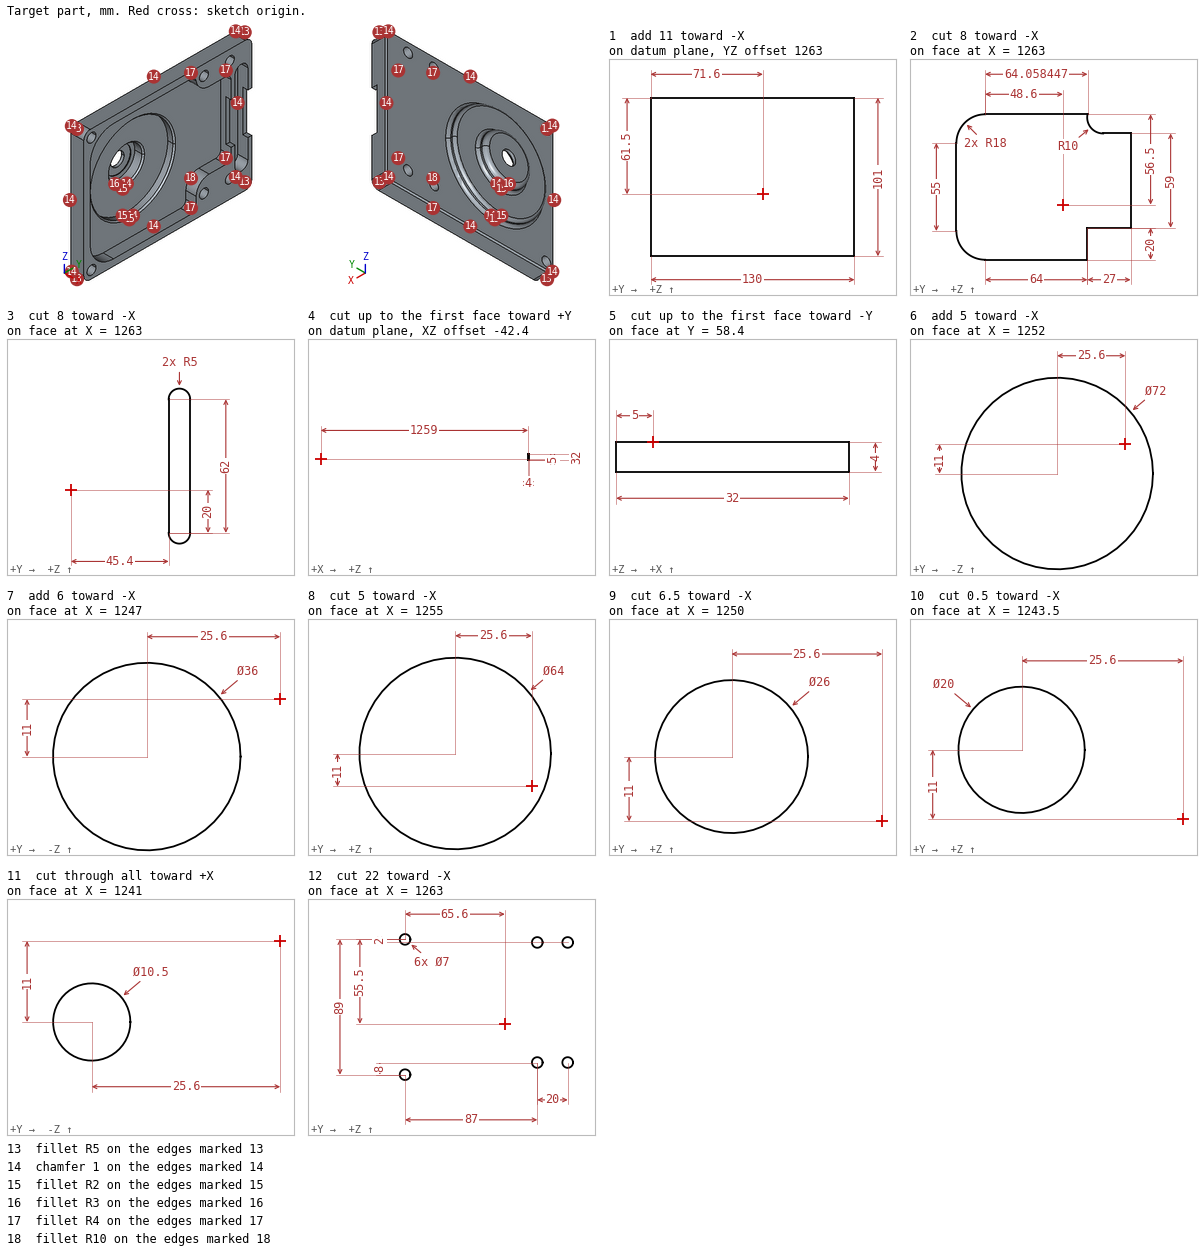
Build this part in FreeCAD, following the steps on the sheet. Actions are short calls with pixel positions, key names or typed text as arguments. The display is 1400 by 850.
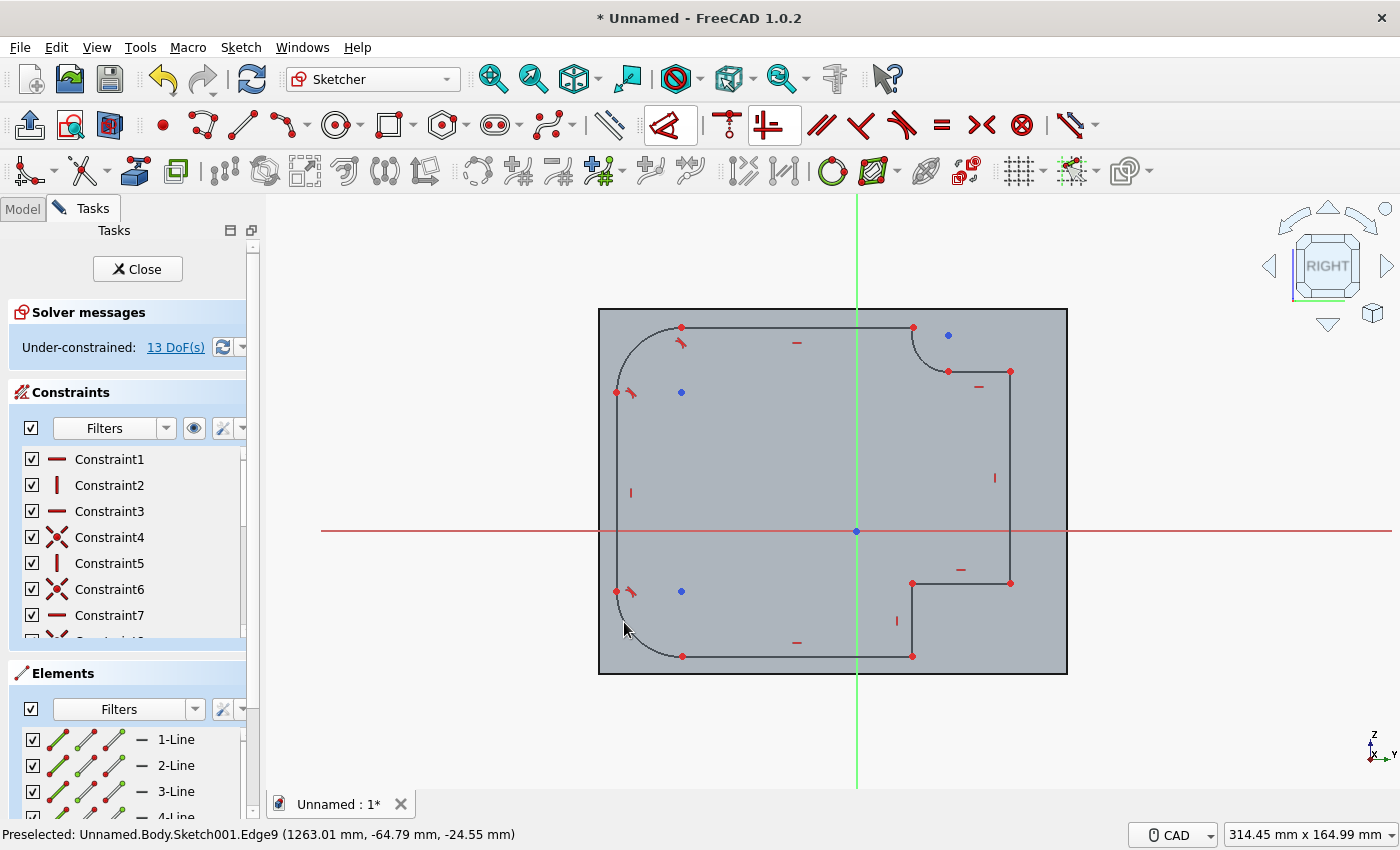
click(751, 657)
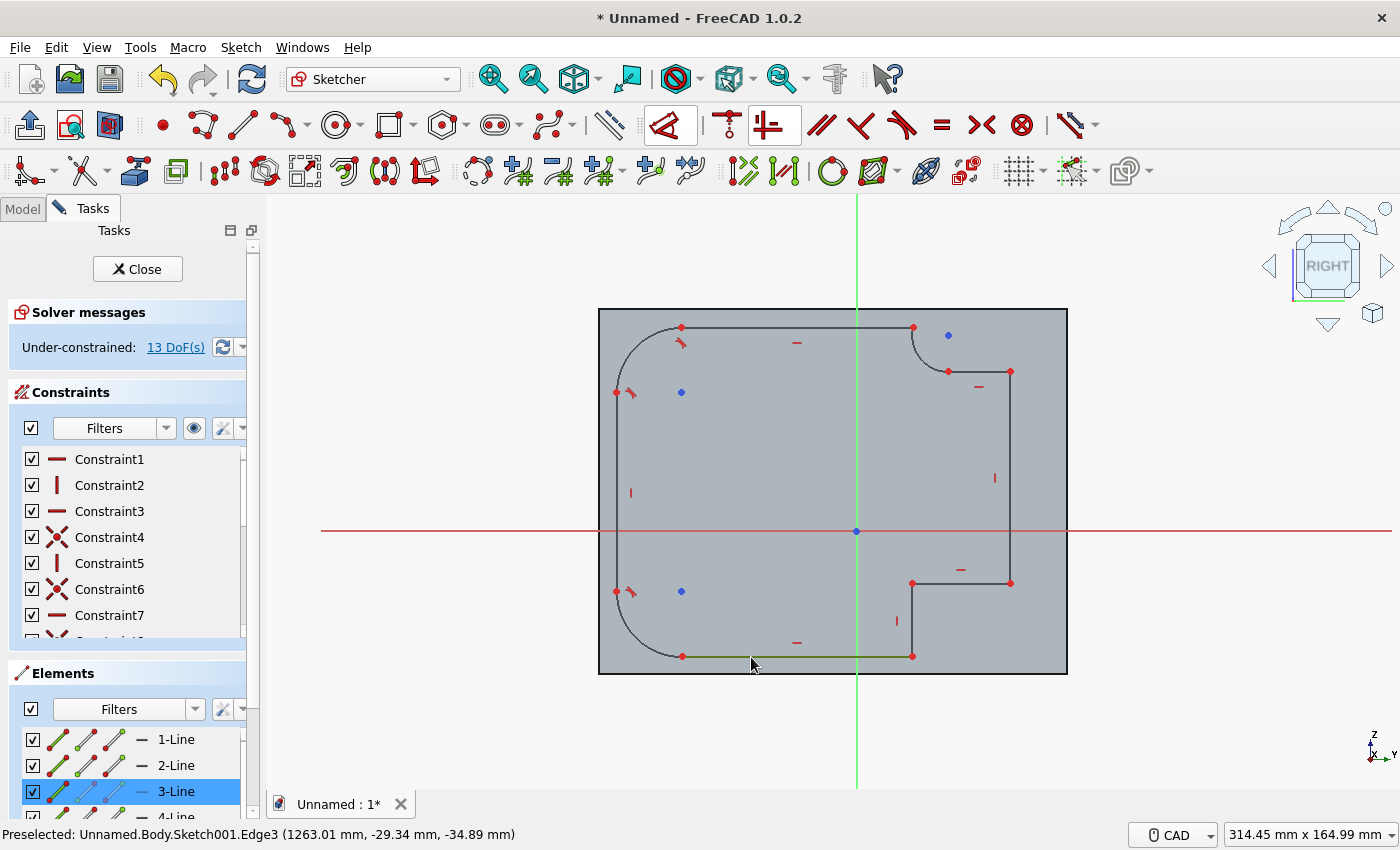
click(624, 622)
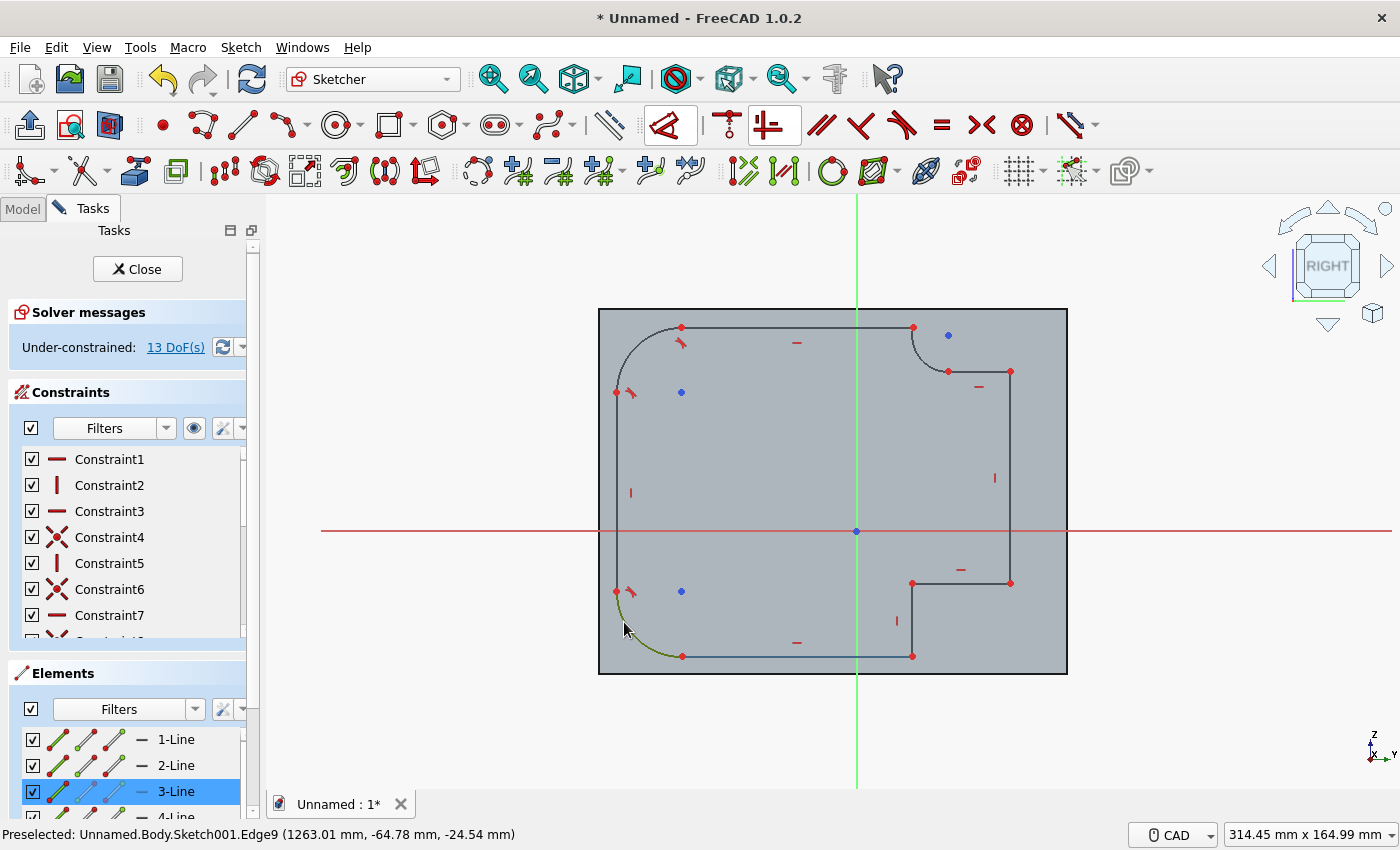
key(t)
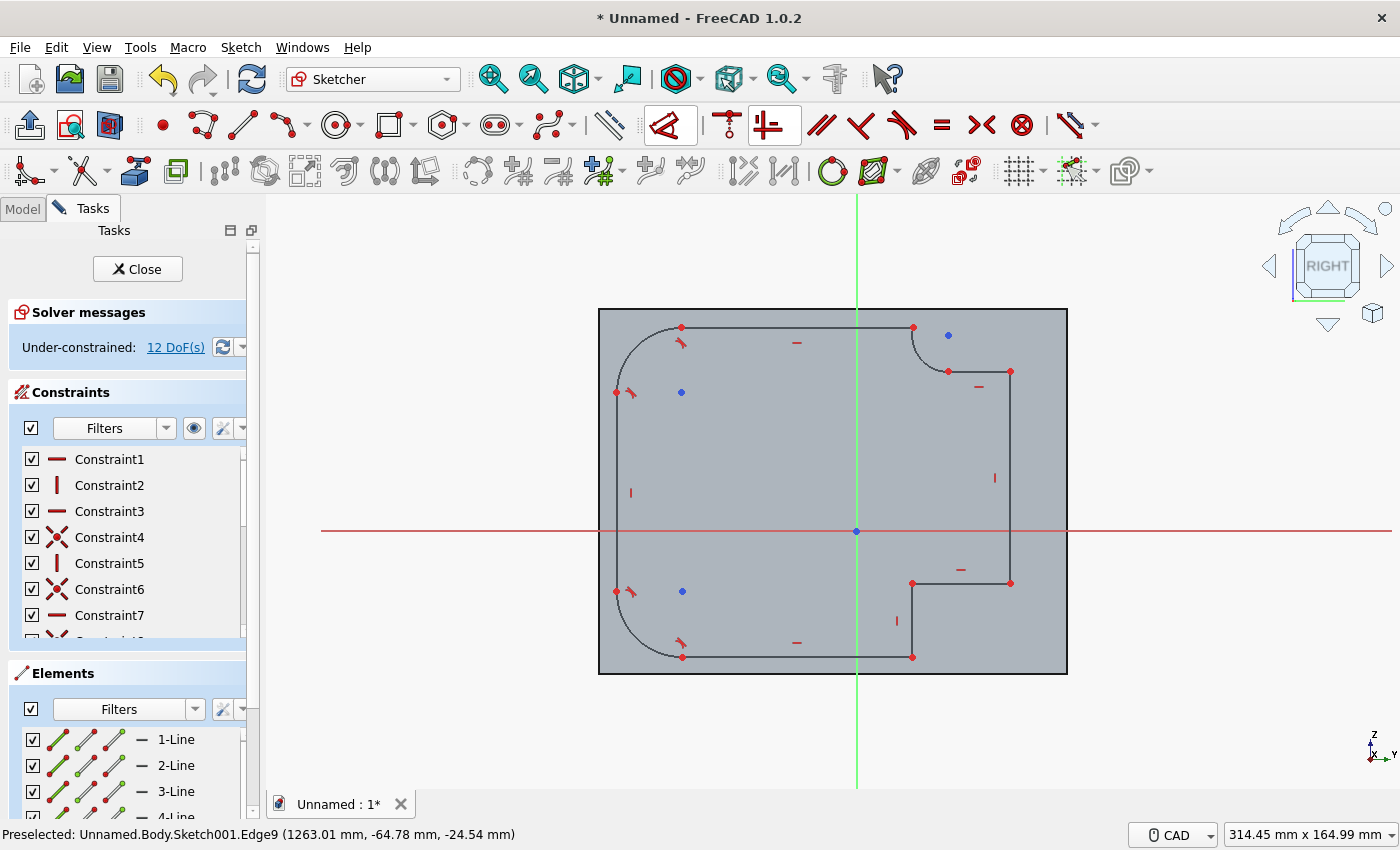
click(991, 372)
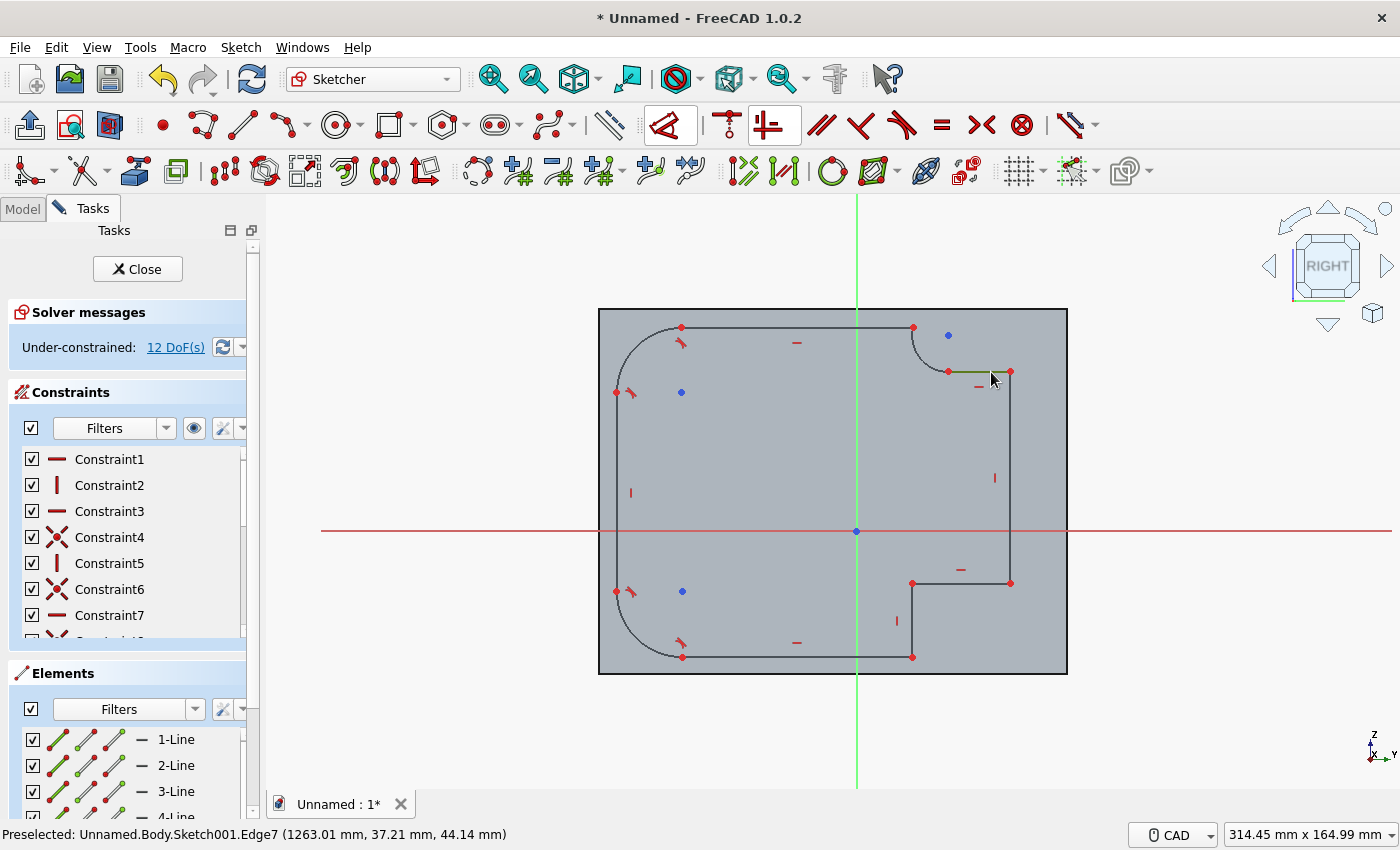
click(914, 347)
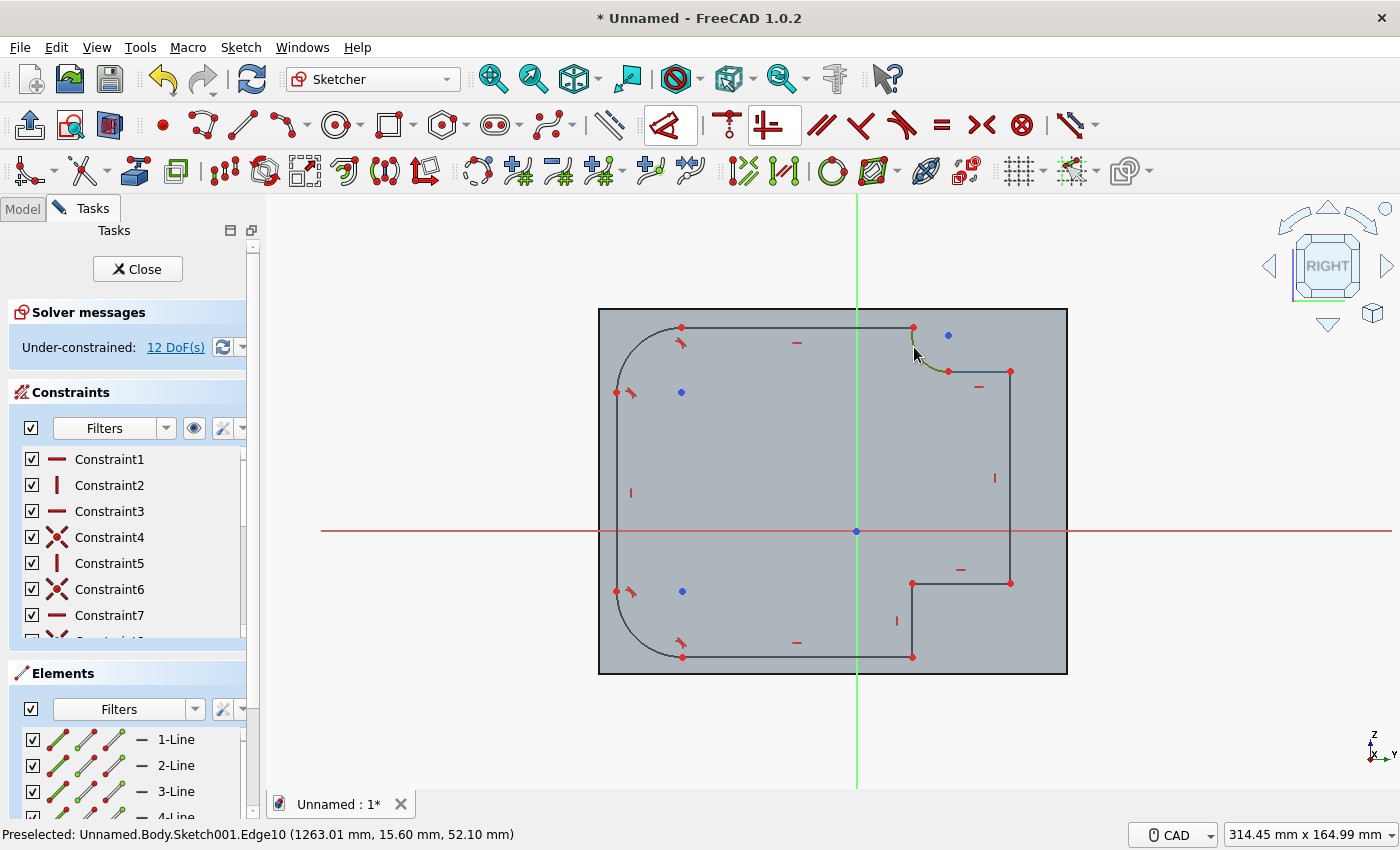
key(t)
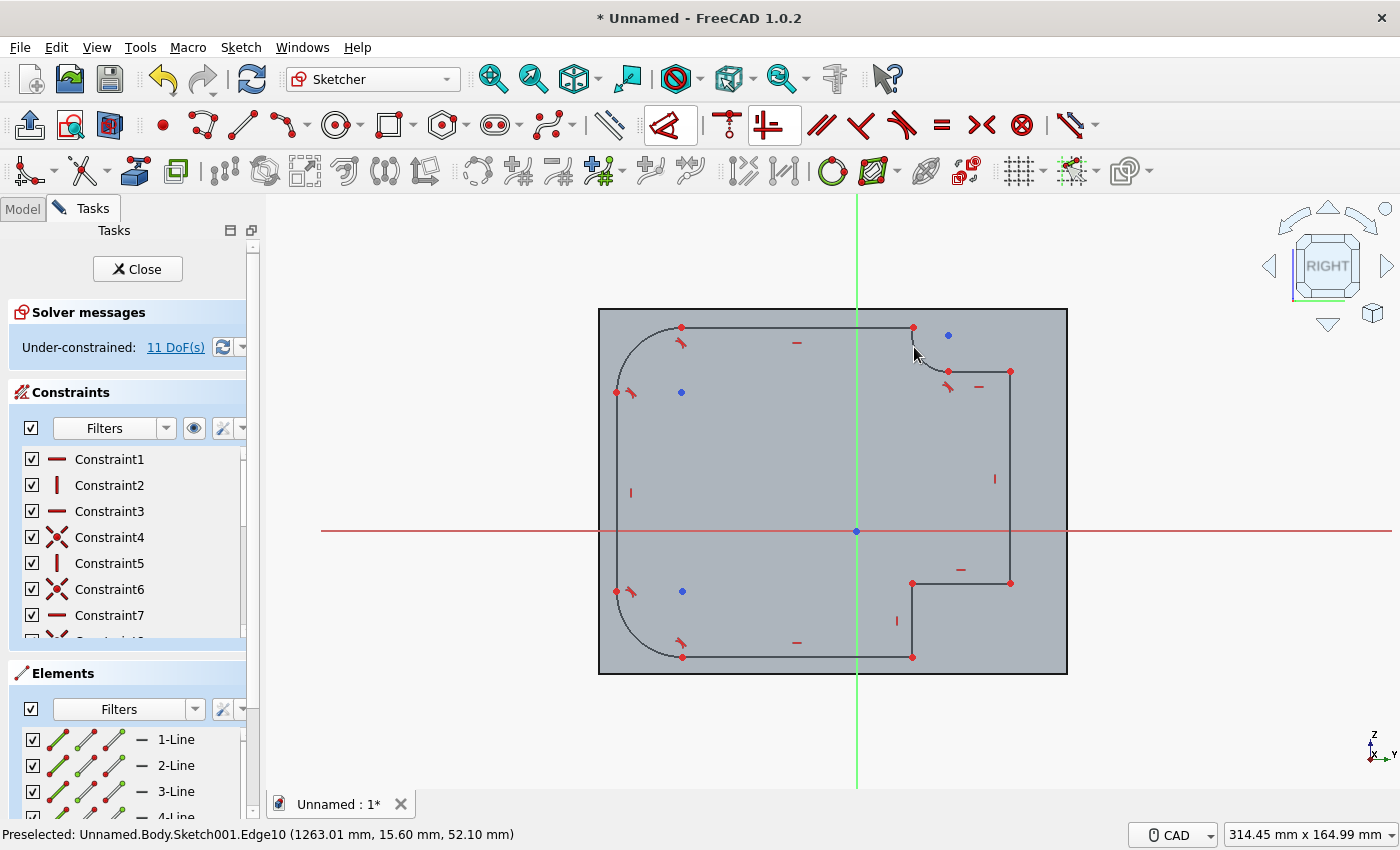
click(652, 335)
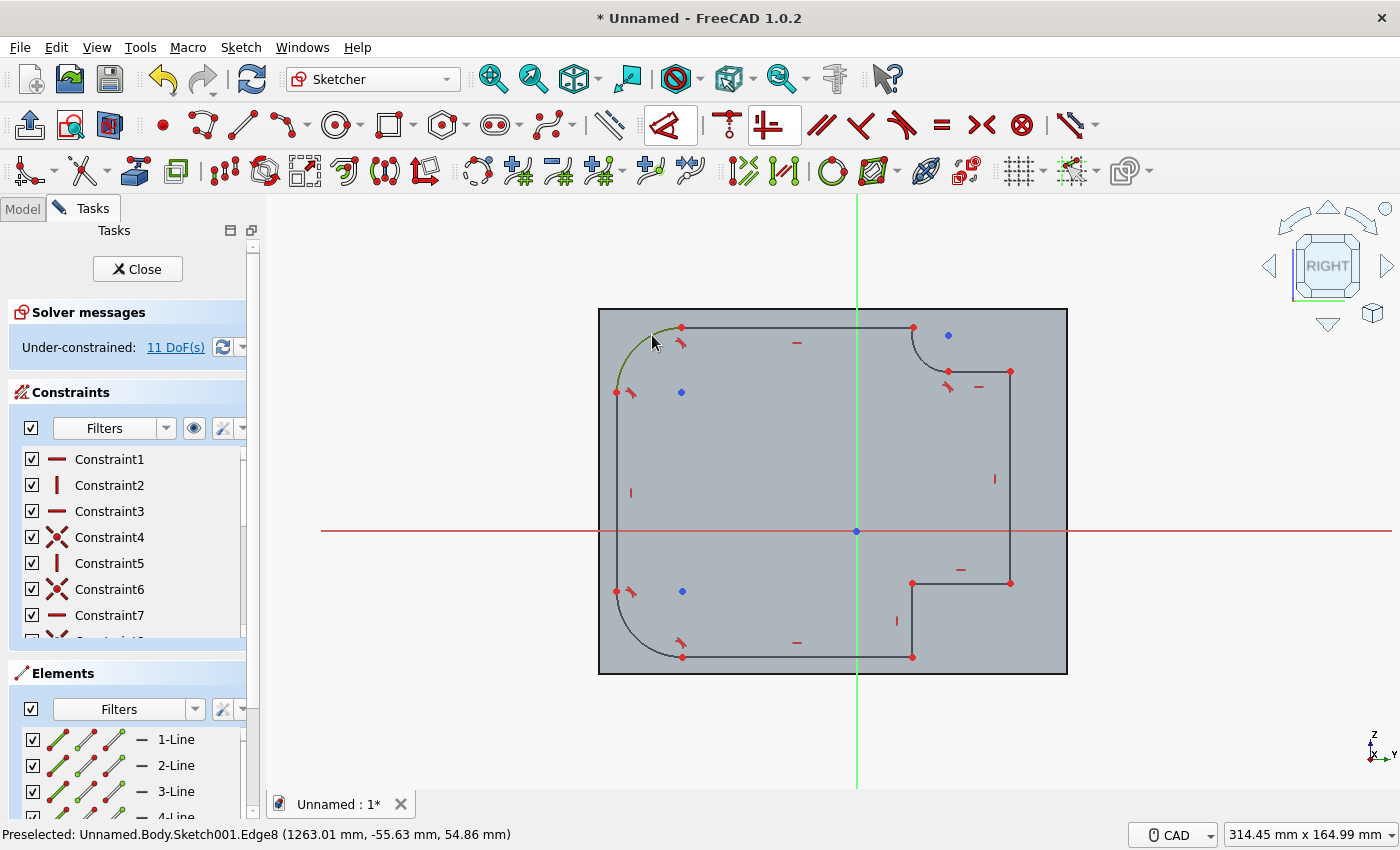
click(624, 622)